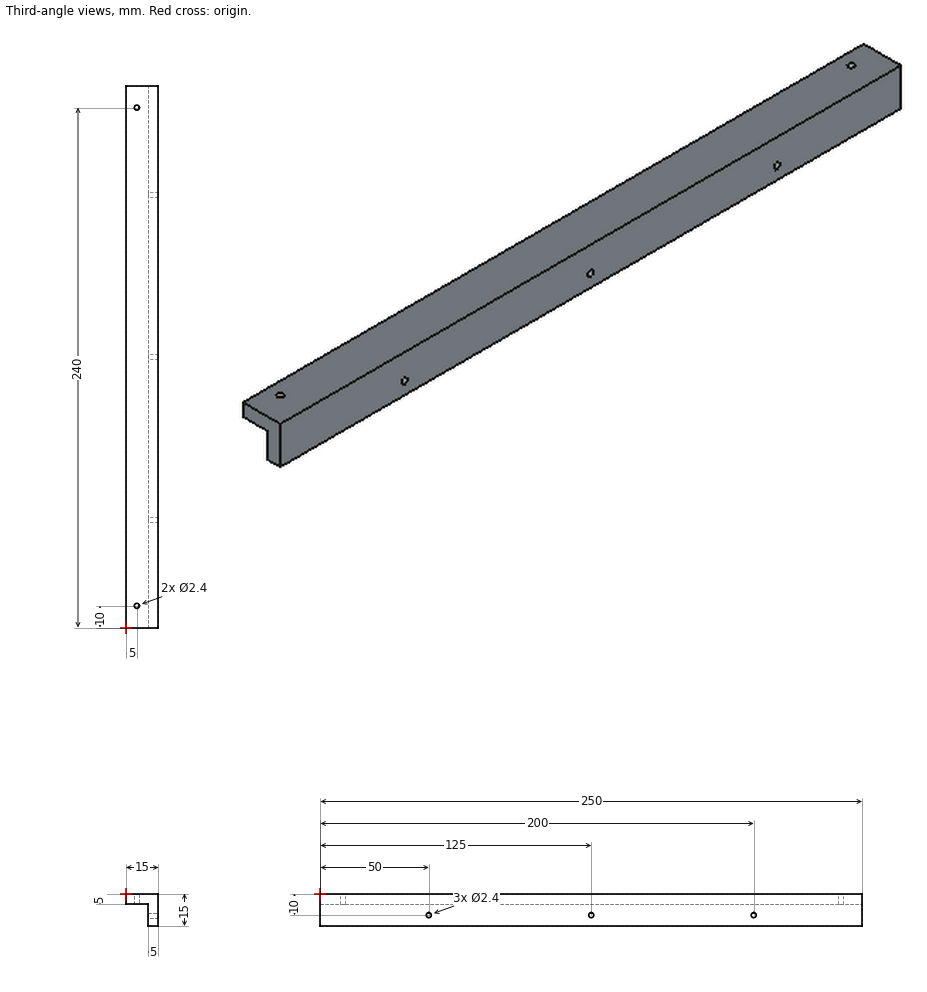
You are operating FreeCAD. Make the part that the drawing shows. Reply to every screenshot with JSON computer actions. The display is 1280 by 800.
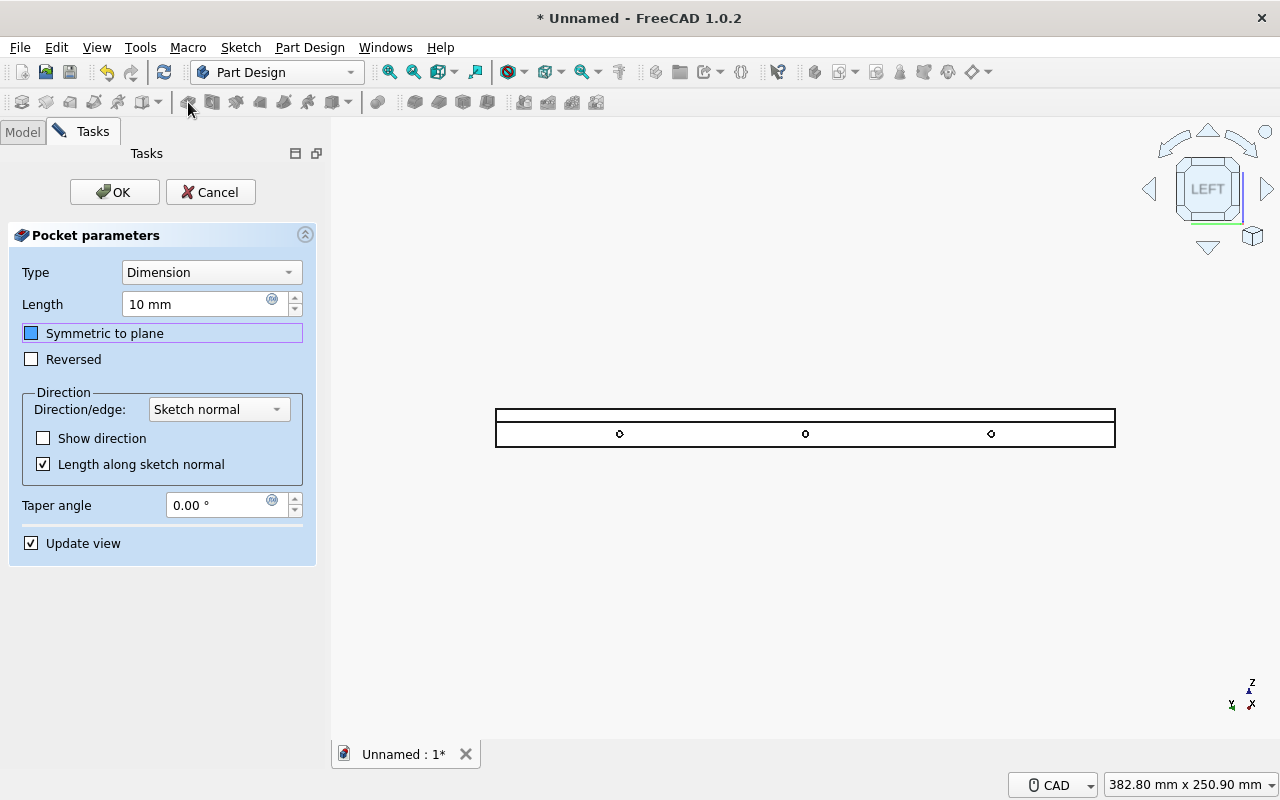
{"action": "left_click", "coordinate": [115, 192]}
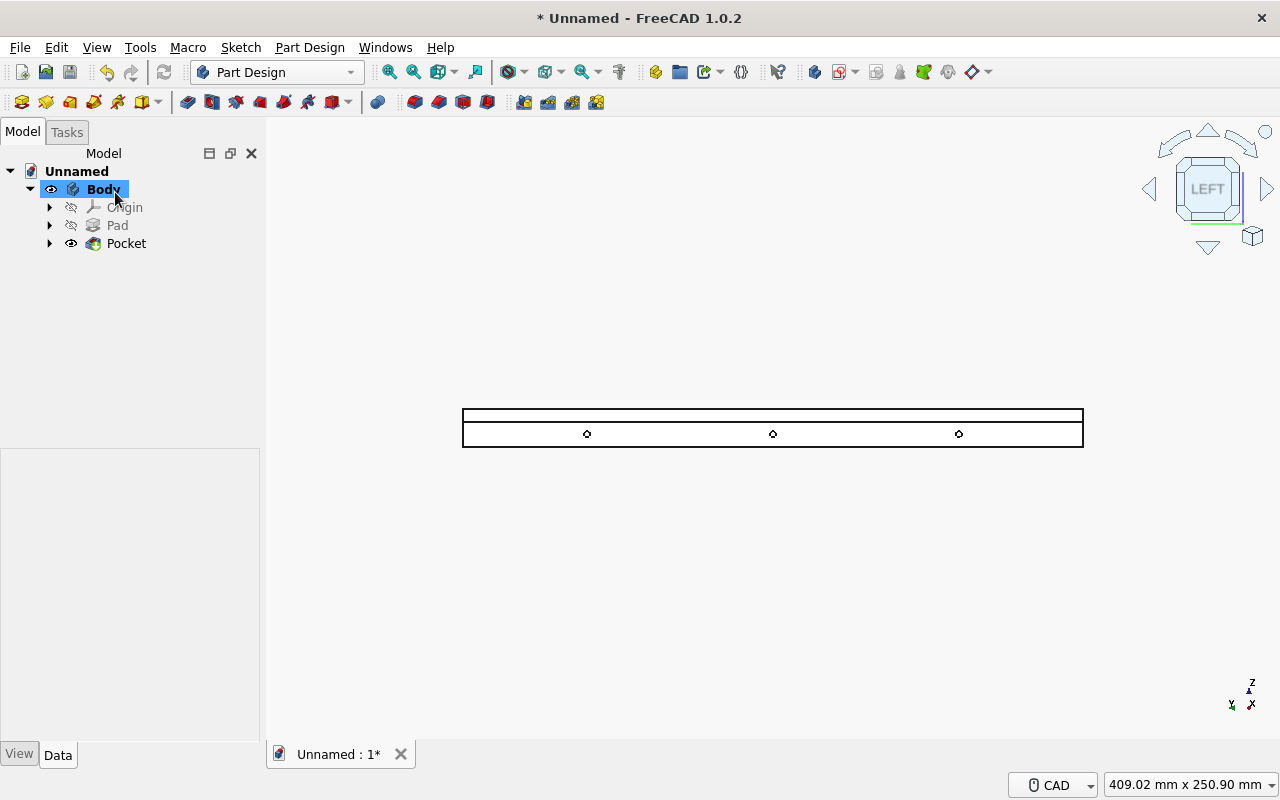
{"action": "left_click", "coordinate": [840, 72]}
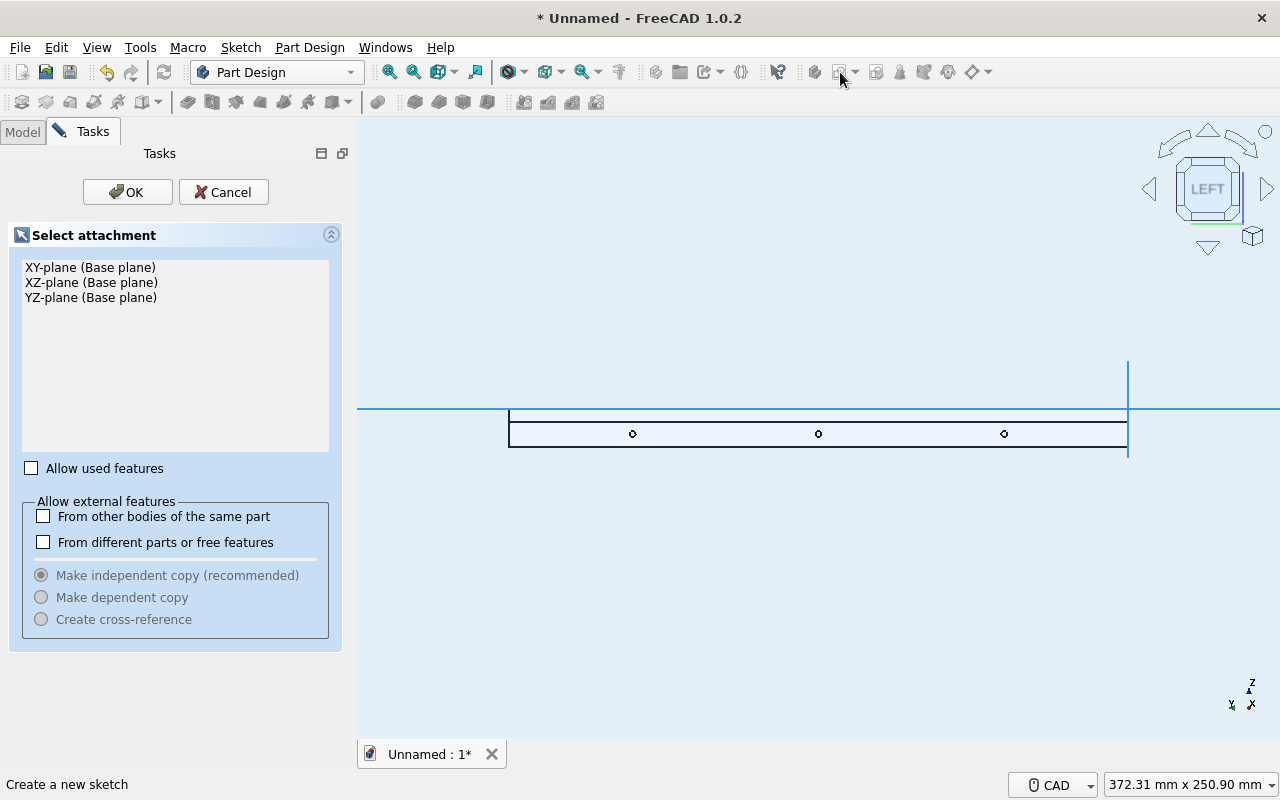
{"action": "left_click", "coordinate": [82, 268]}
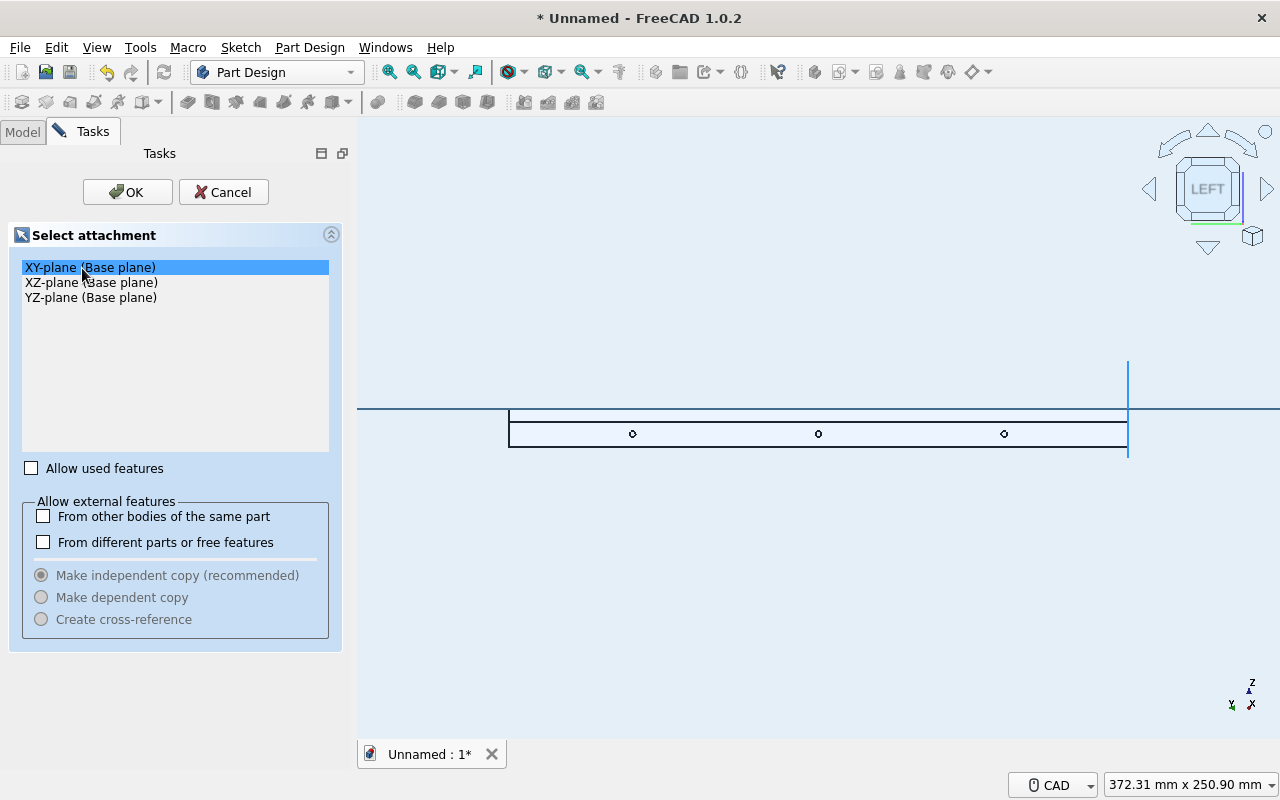
{"action": "left_click", "coordinate": [128, 192]}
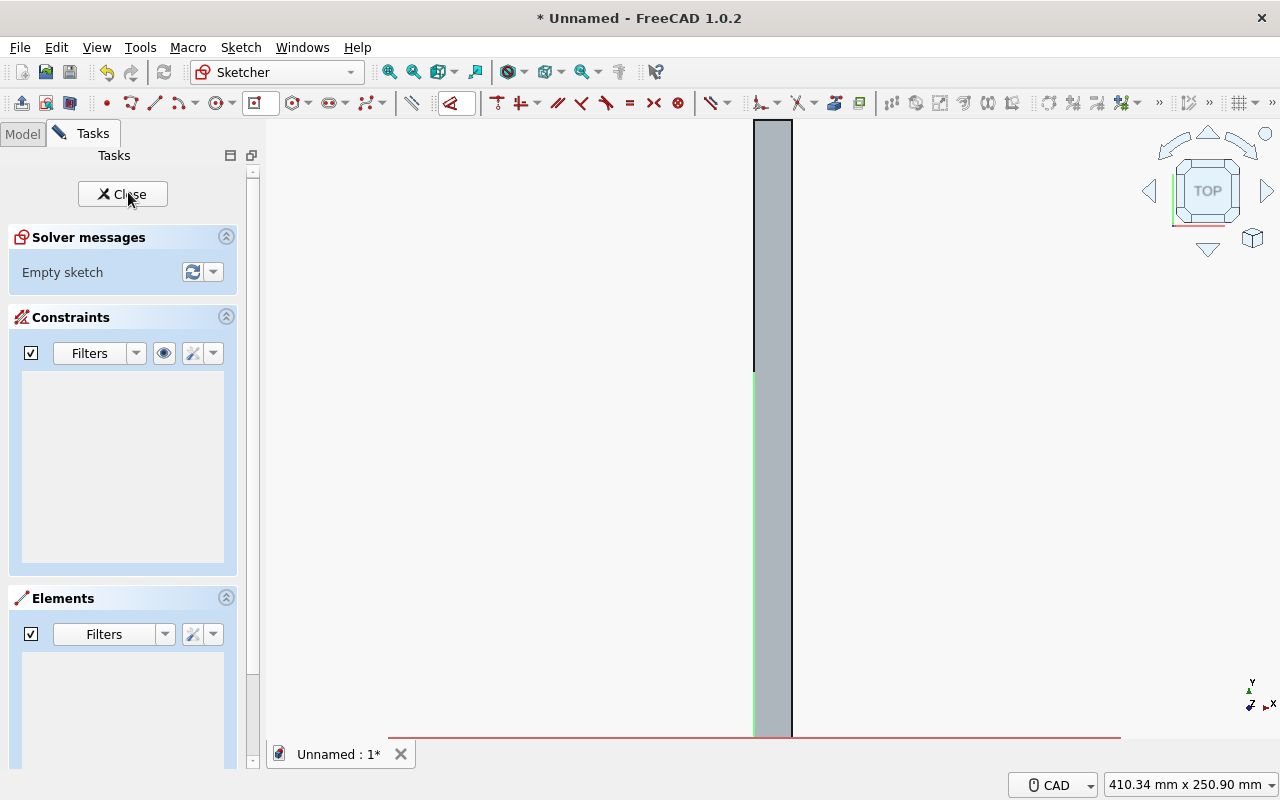
{"action": "scroll", "coordinate": [587, 407], "scroll_direction": "down", "scroll_amount": 2}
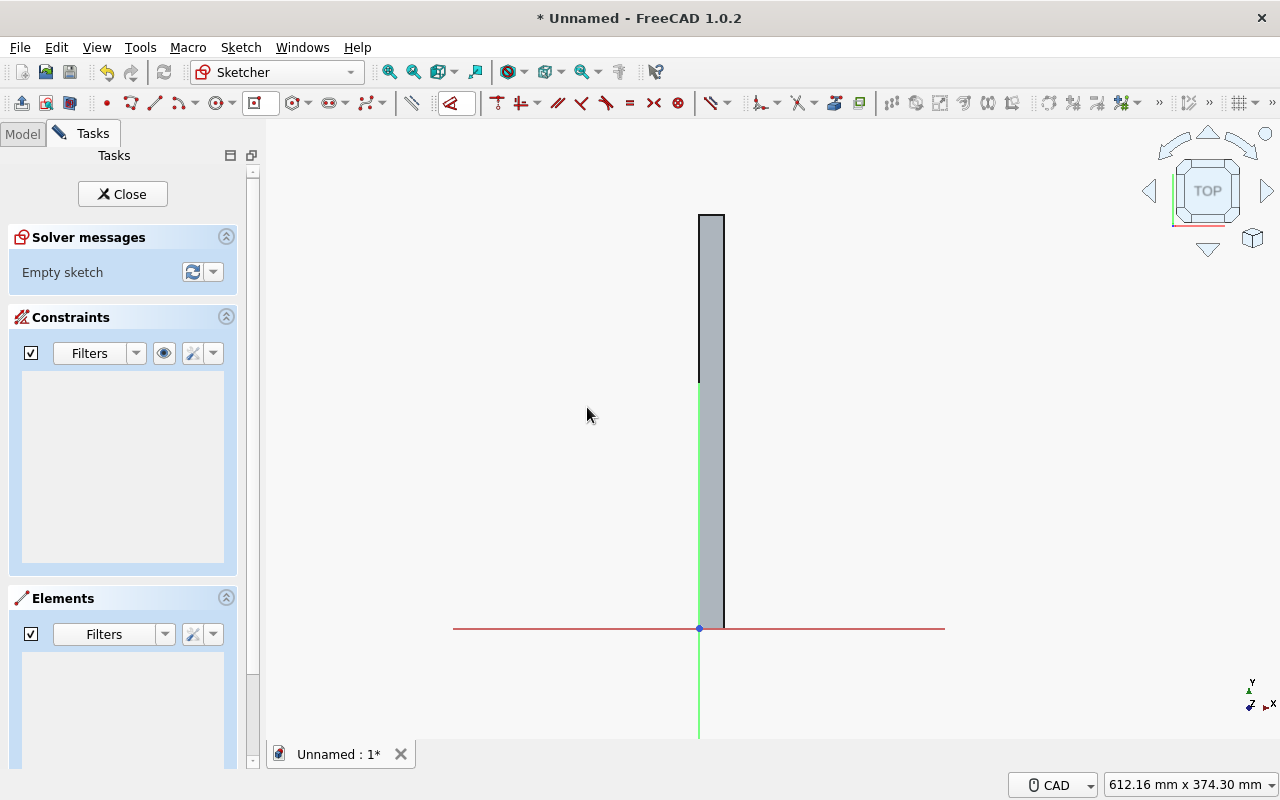
{"action": "key", "text": "g c"}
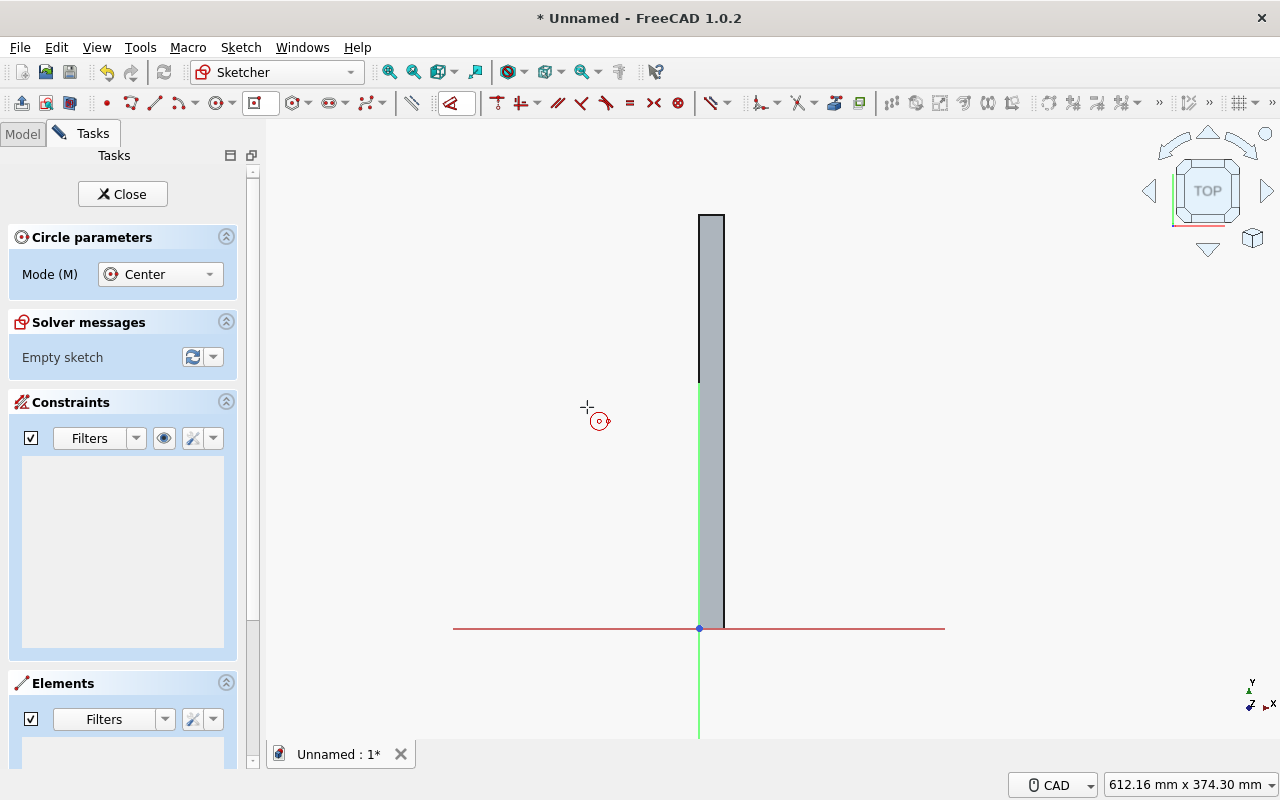
{"action": "scroll", "coordinate": [708, 612], "scroll_direction": "up", "scroll_amount": 13}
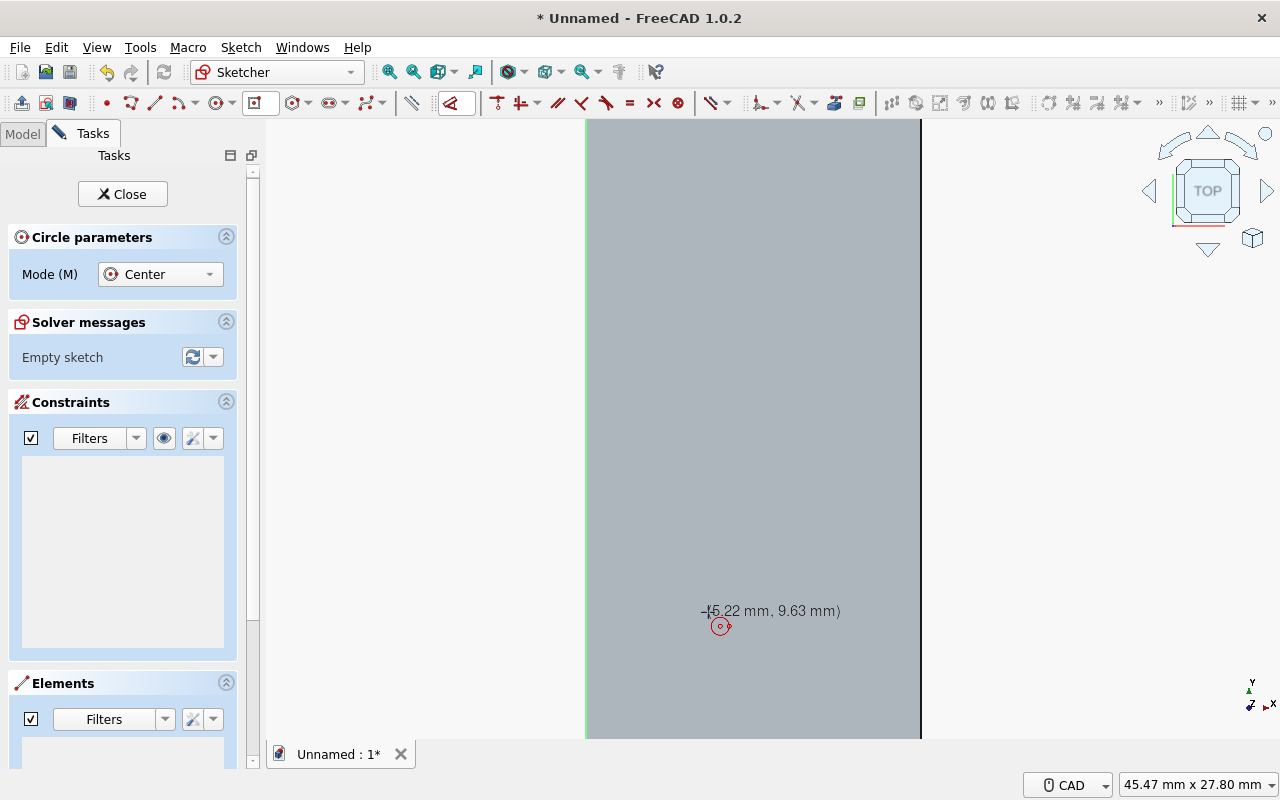
{"action": "scroll", "coordinate": [708, 613], "scroll_direction": "down", "scroll_amount": 13}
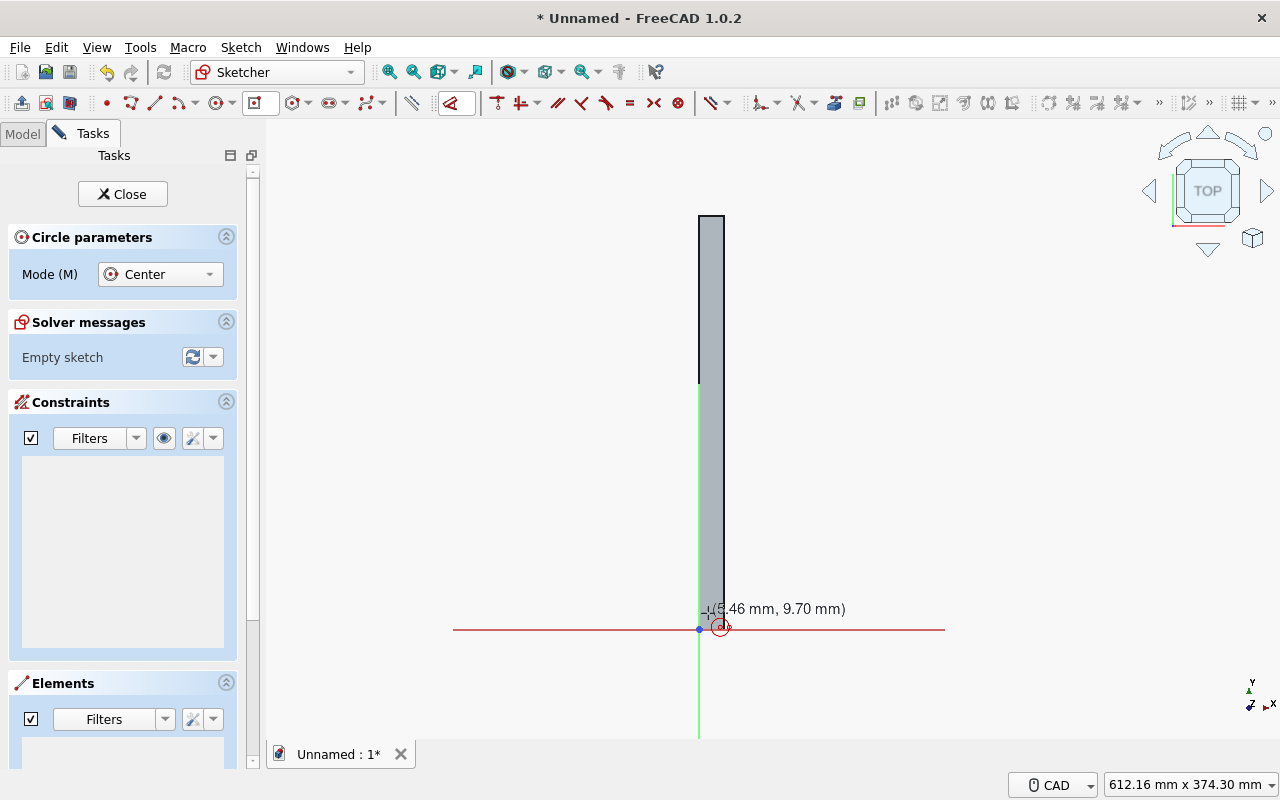
{"action": "scroll", "coordinate": [708, 613], "scroll_direction": "up", "scroll_amount": 4}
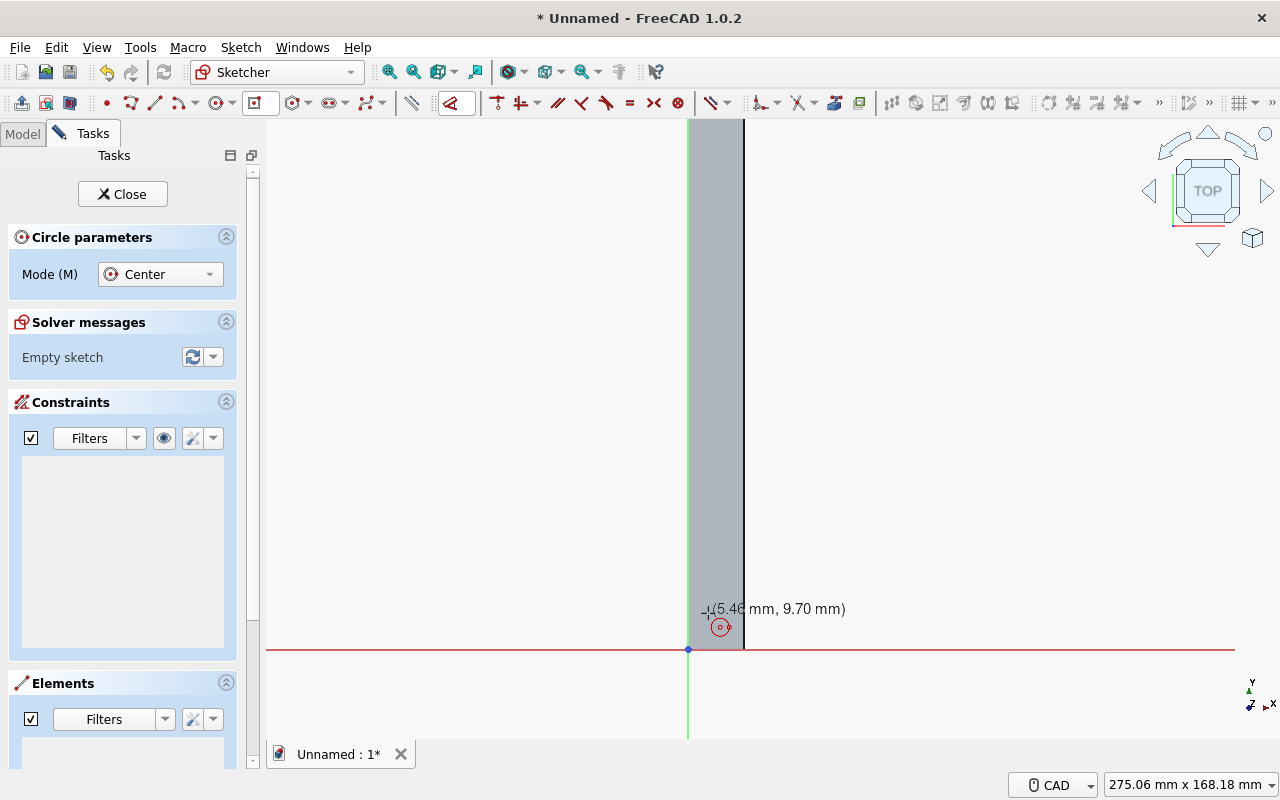
{"action": "left_click", "coordinate": [707, 613]}
{"action": "mouse_move", "coordinate": [710, 610]}